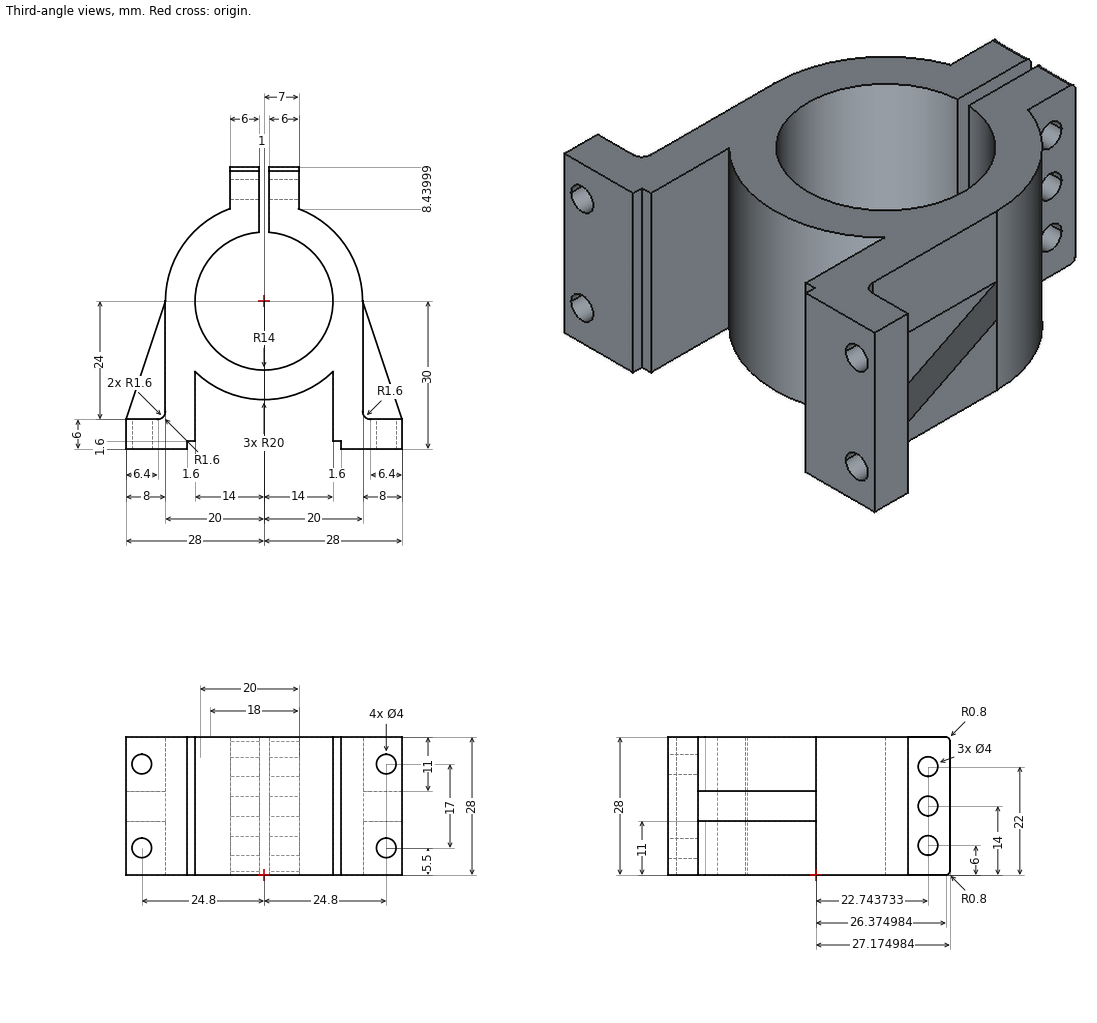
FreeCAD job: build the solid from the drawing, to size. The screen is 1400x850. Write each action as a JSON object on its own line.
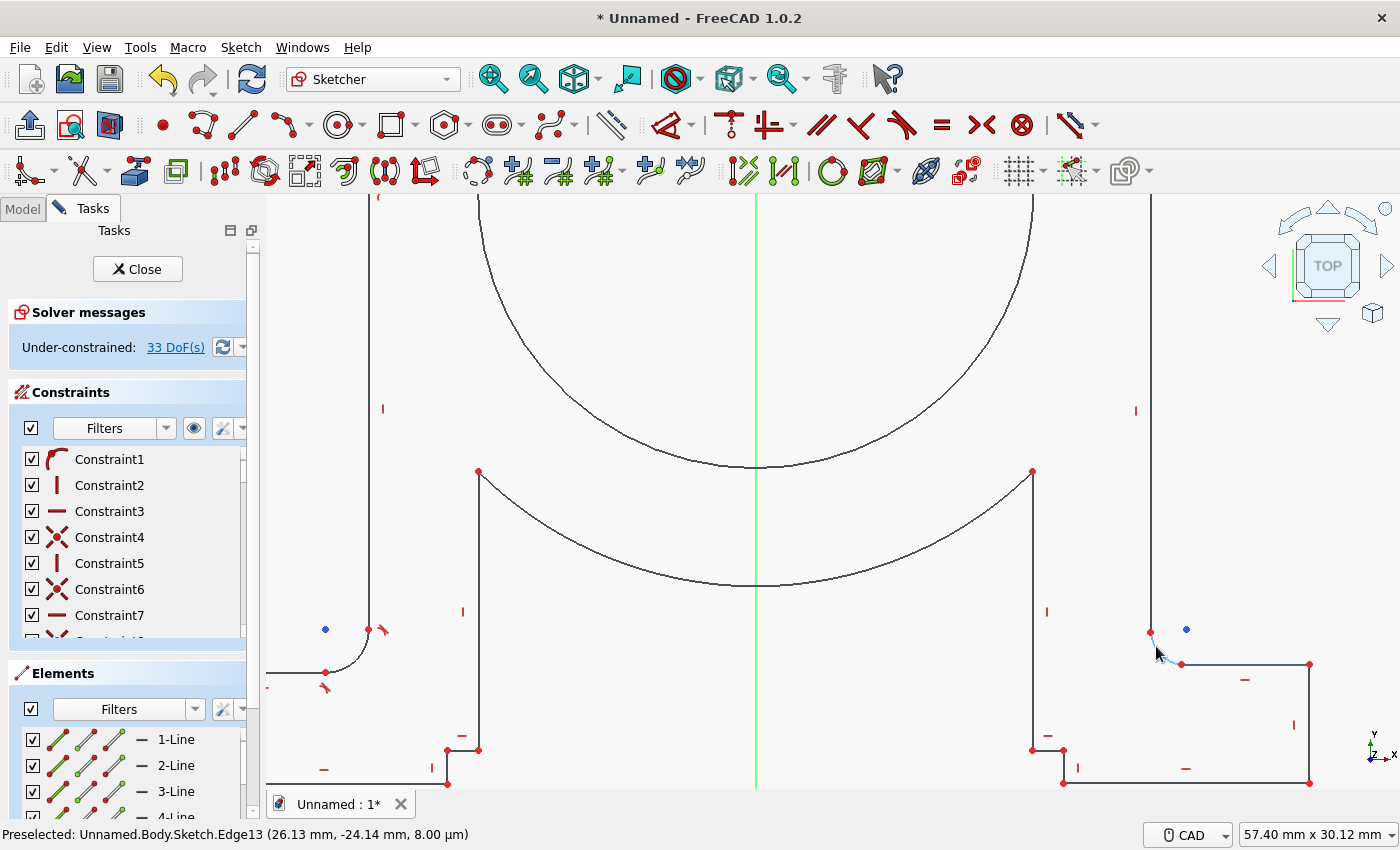
{"action": "left_click", "coordinate": [1155, 646]}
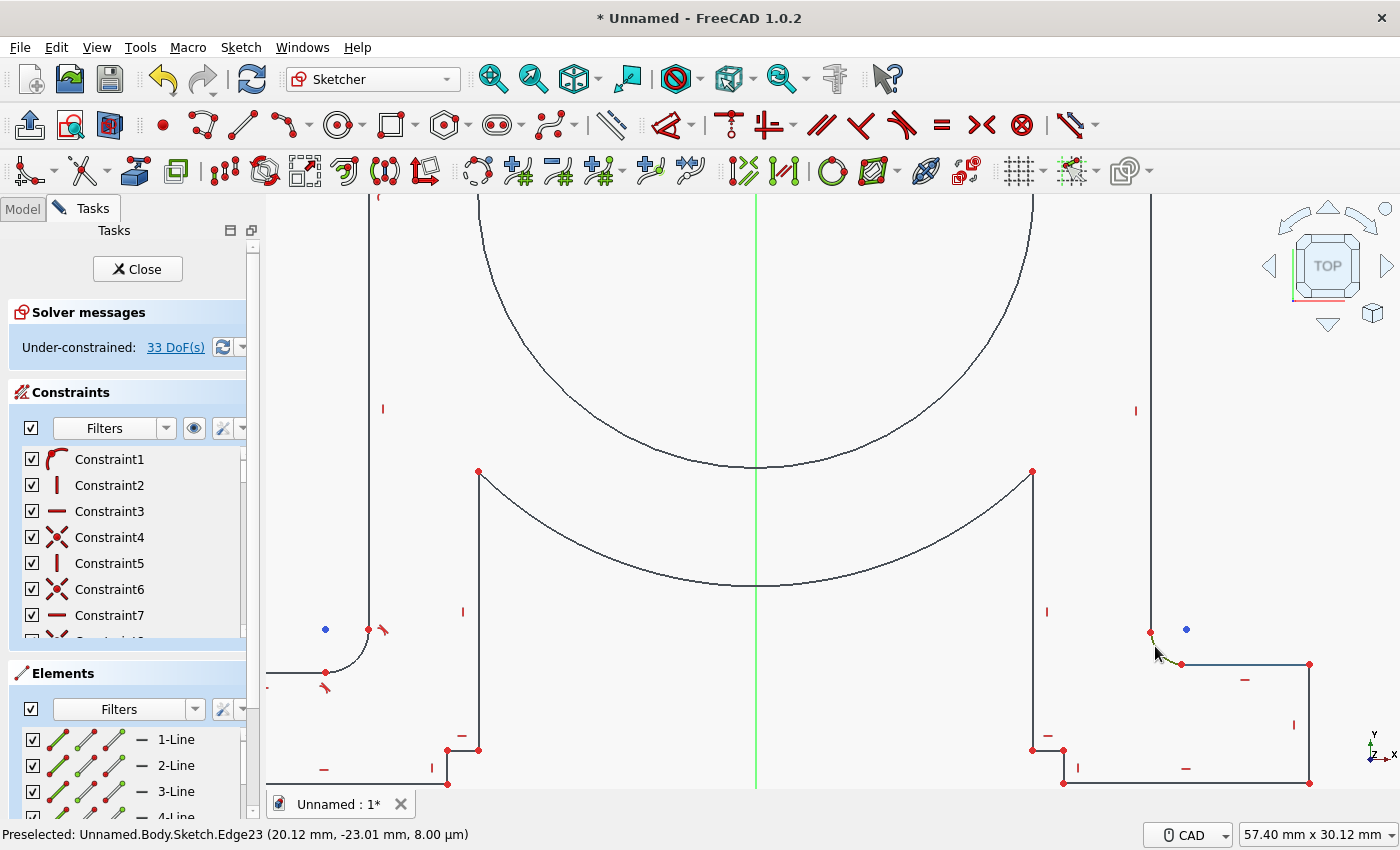
{"action": "left_click", "coordinate": [902, 126]}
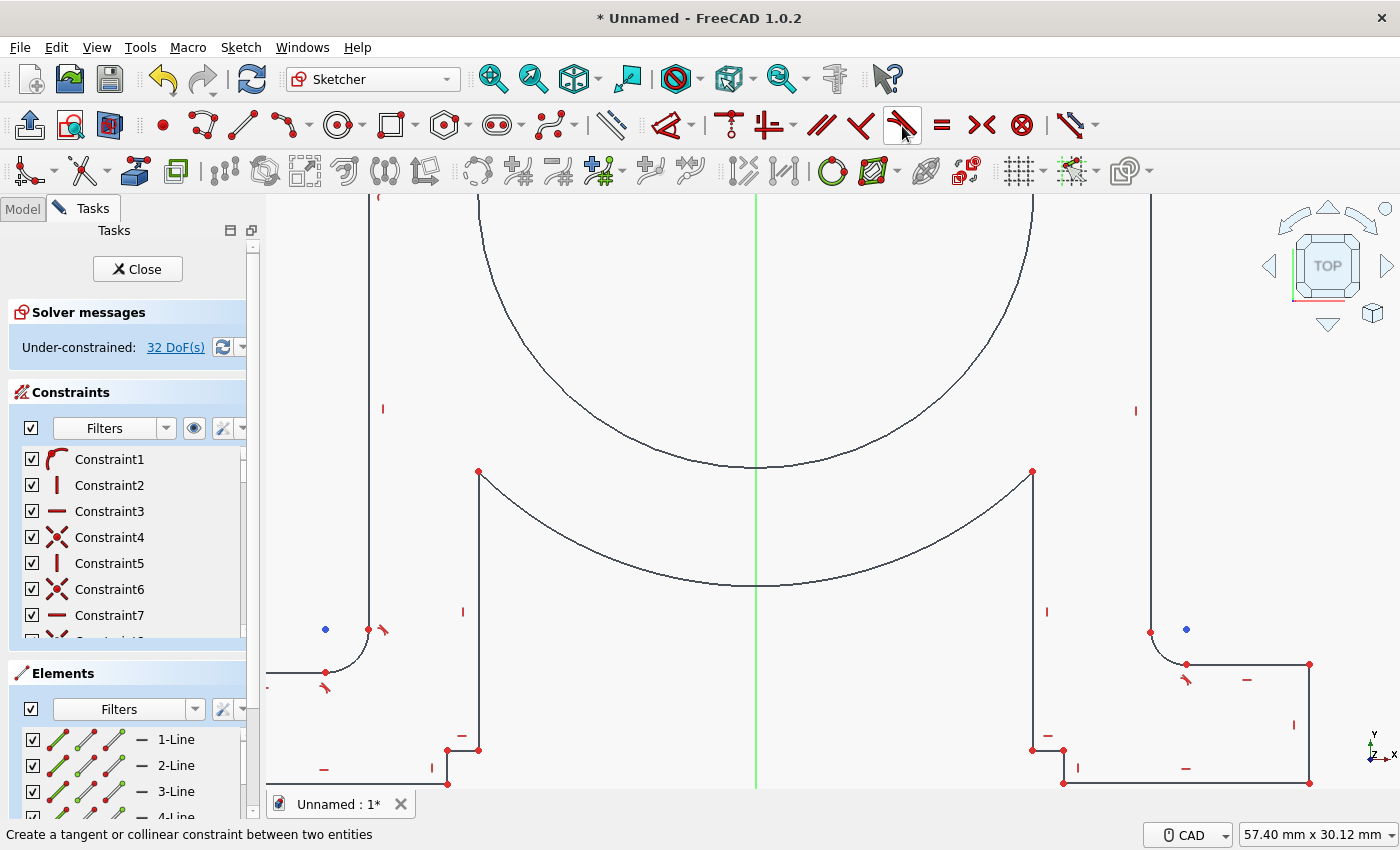
{"action": "left_click", "coordinate": [1151, 499]}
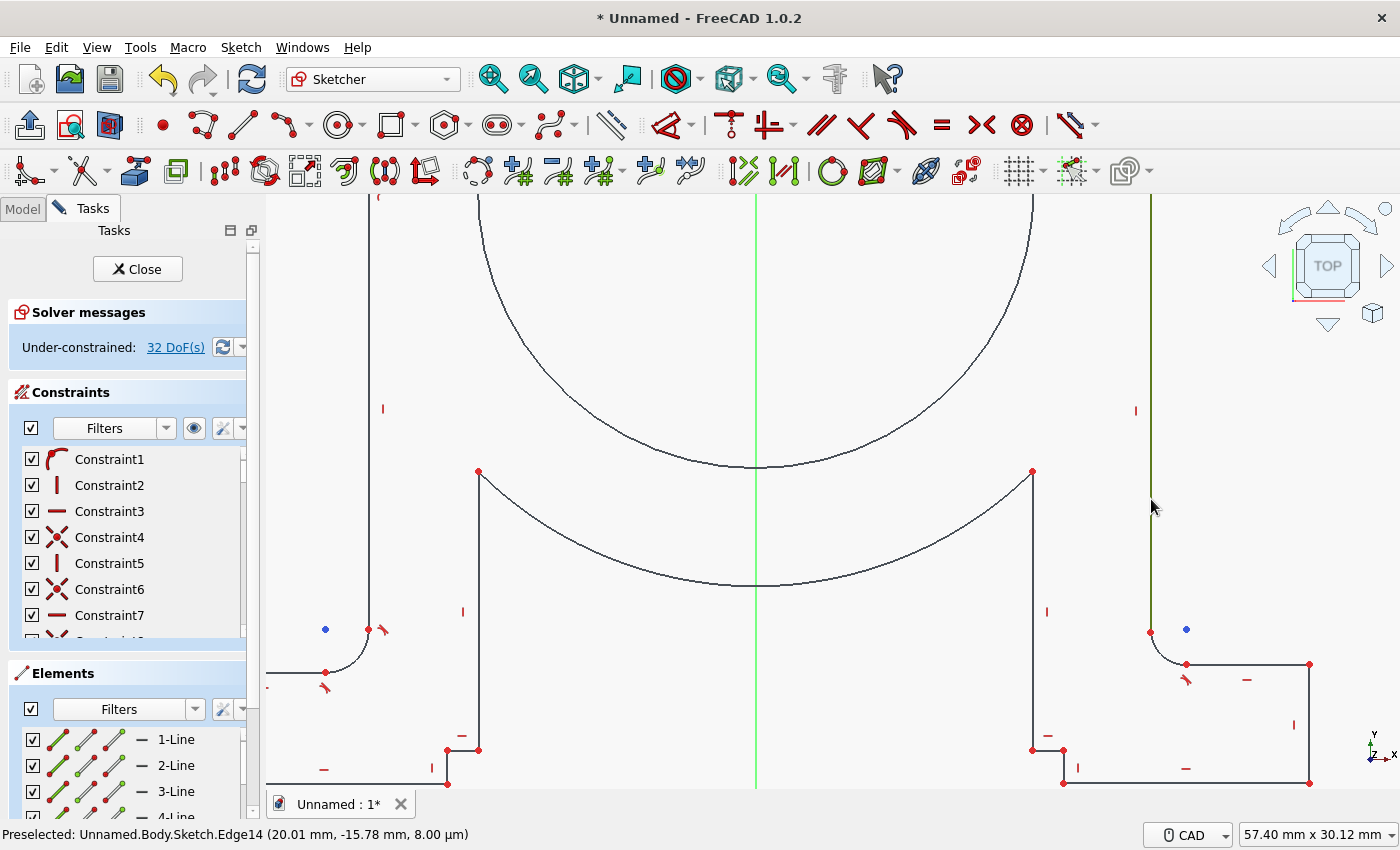
{"action": "left_click", "coordinate": [1156, 647]}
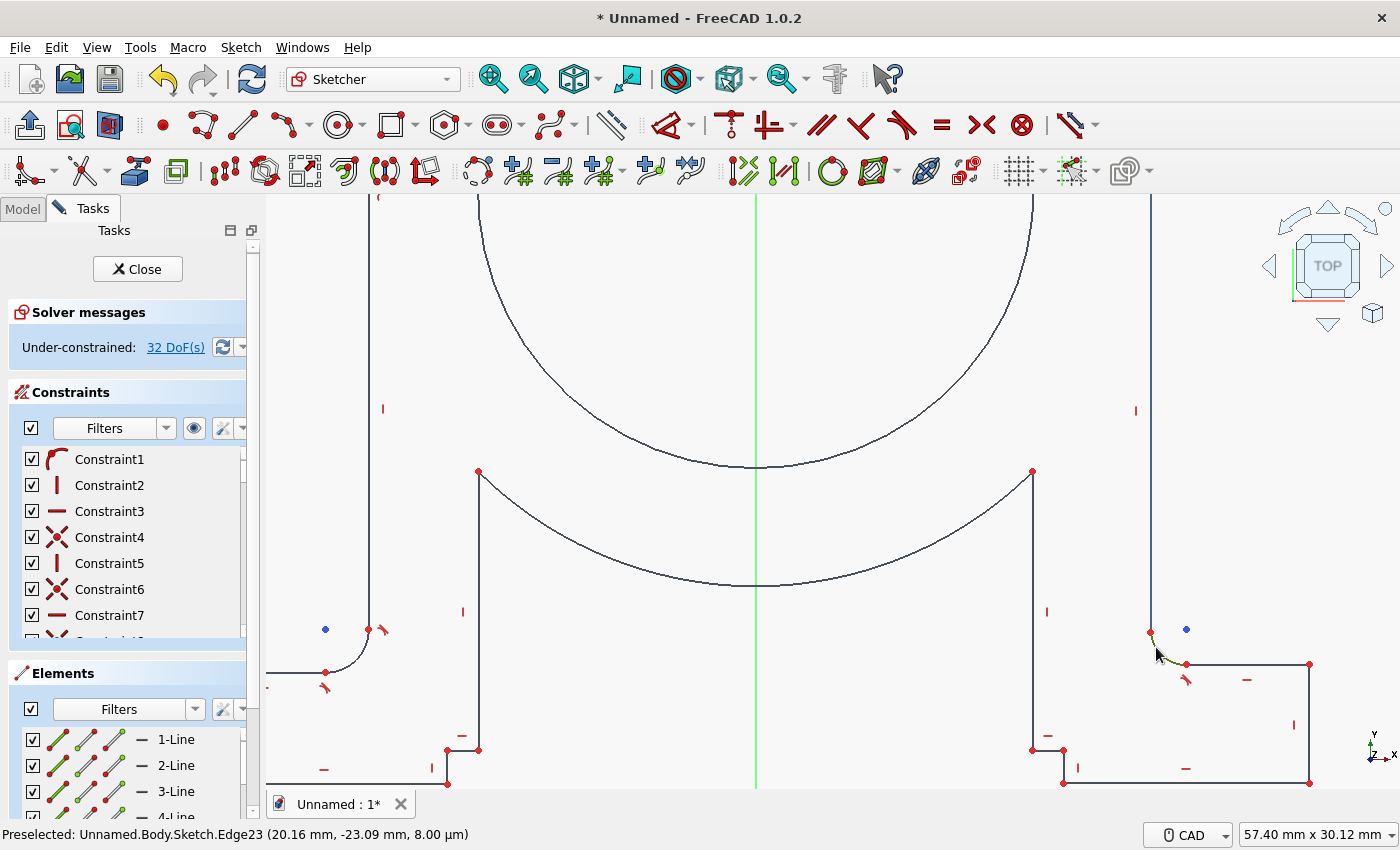
{"action": "left_click", "coordinate": [902, 126]}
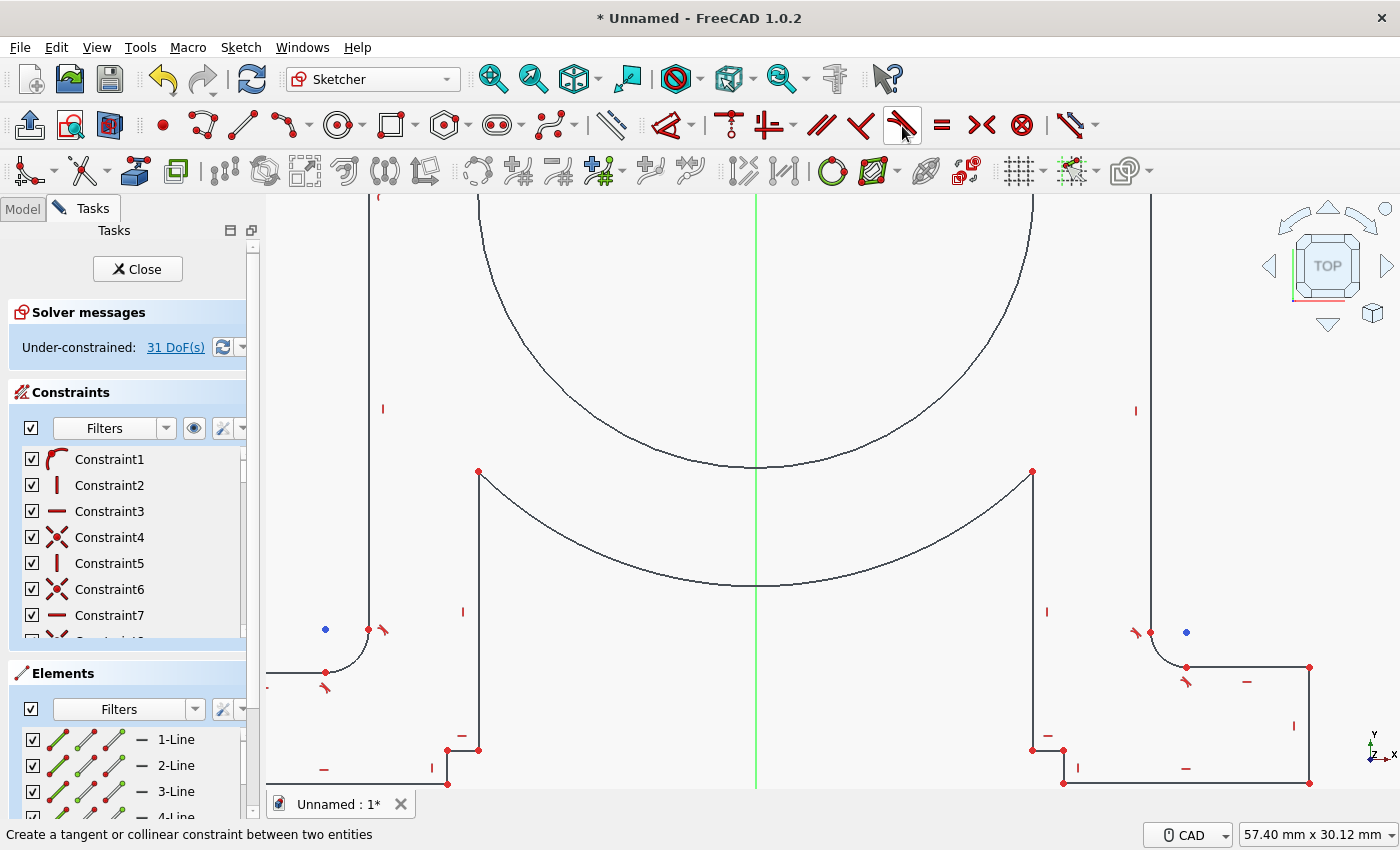
{"action": "left_click", "coordinate": [1151, 499]}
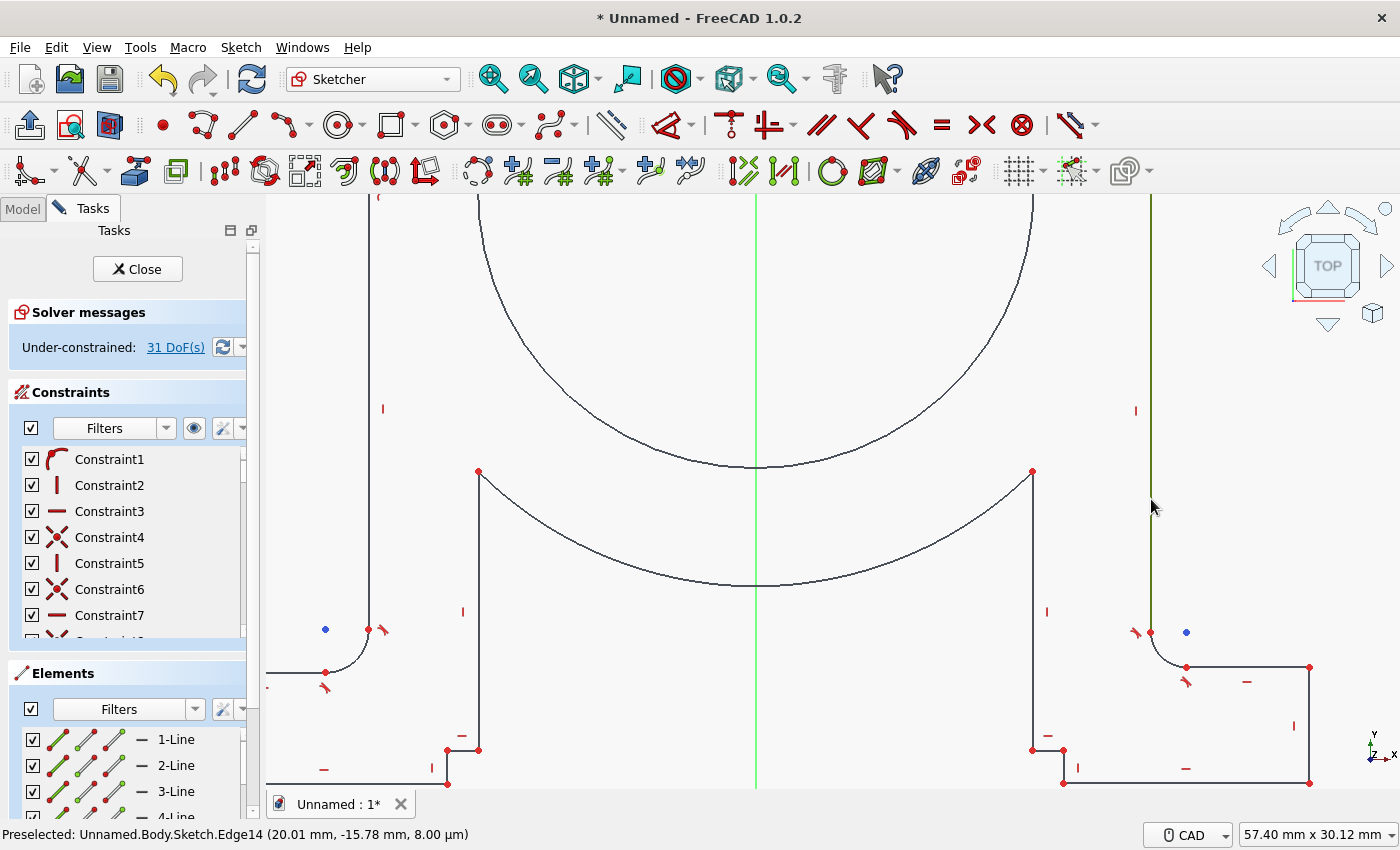
{"action": "scroll", "coordinate": [770, 652], "scroll_direction": "down", "scroll_amount": 5}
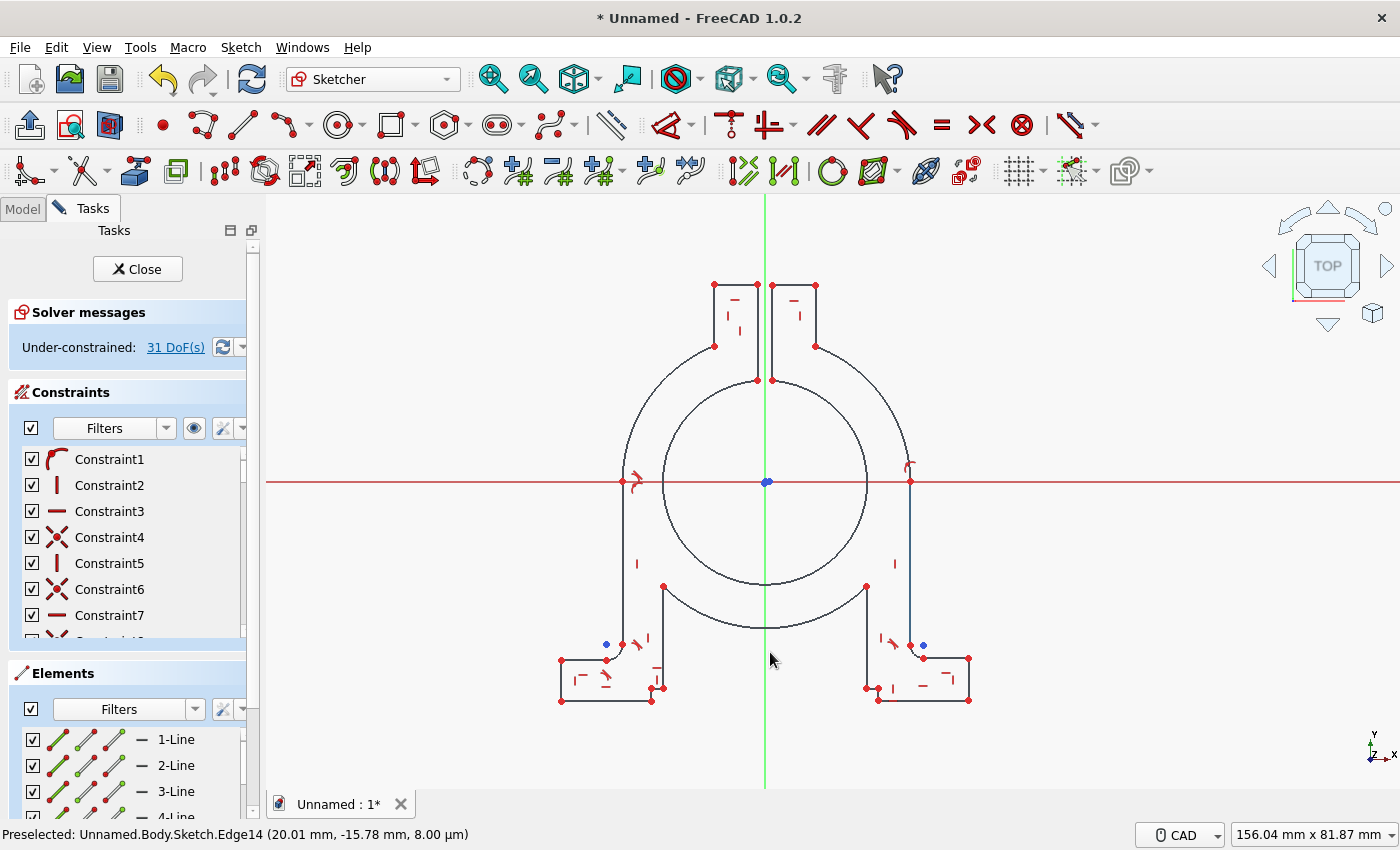
{"action": "left_click", "coordinate": [901, 430]}